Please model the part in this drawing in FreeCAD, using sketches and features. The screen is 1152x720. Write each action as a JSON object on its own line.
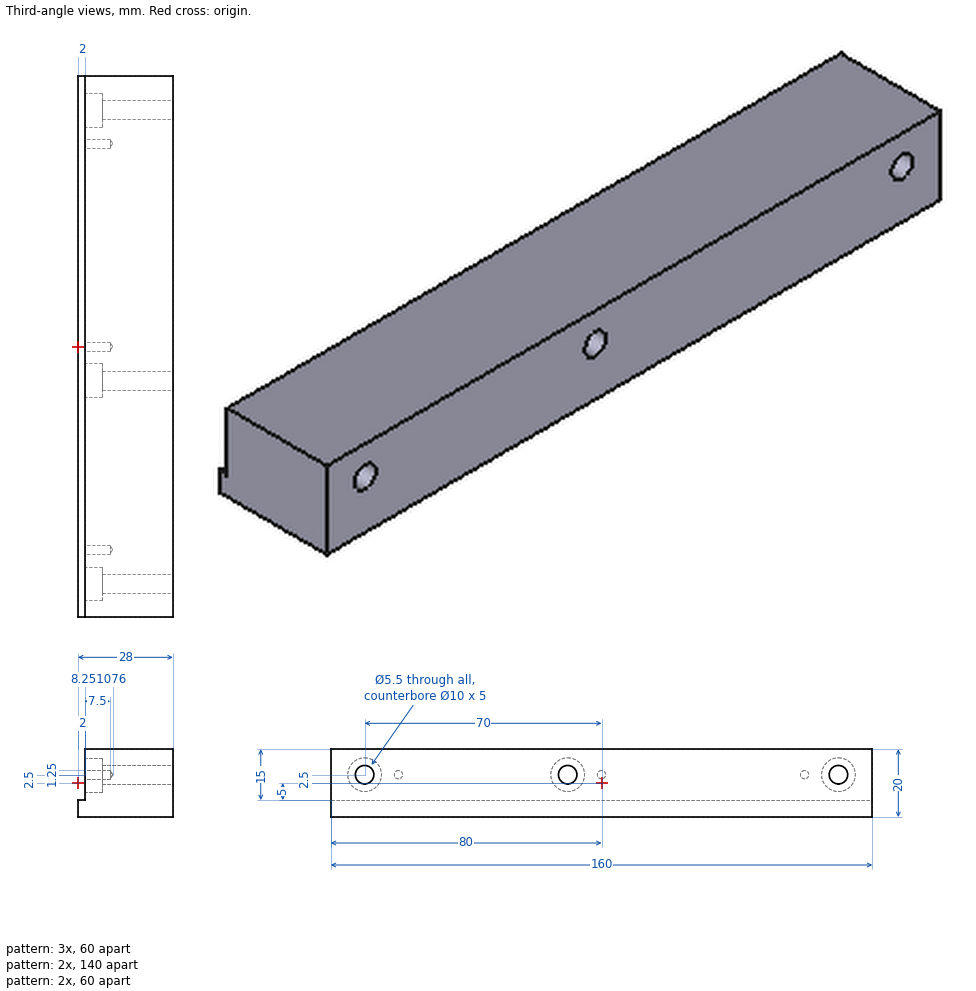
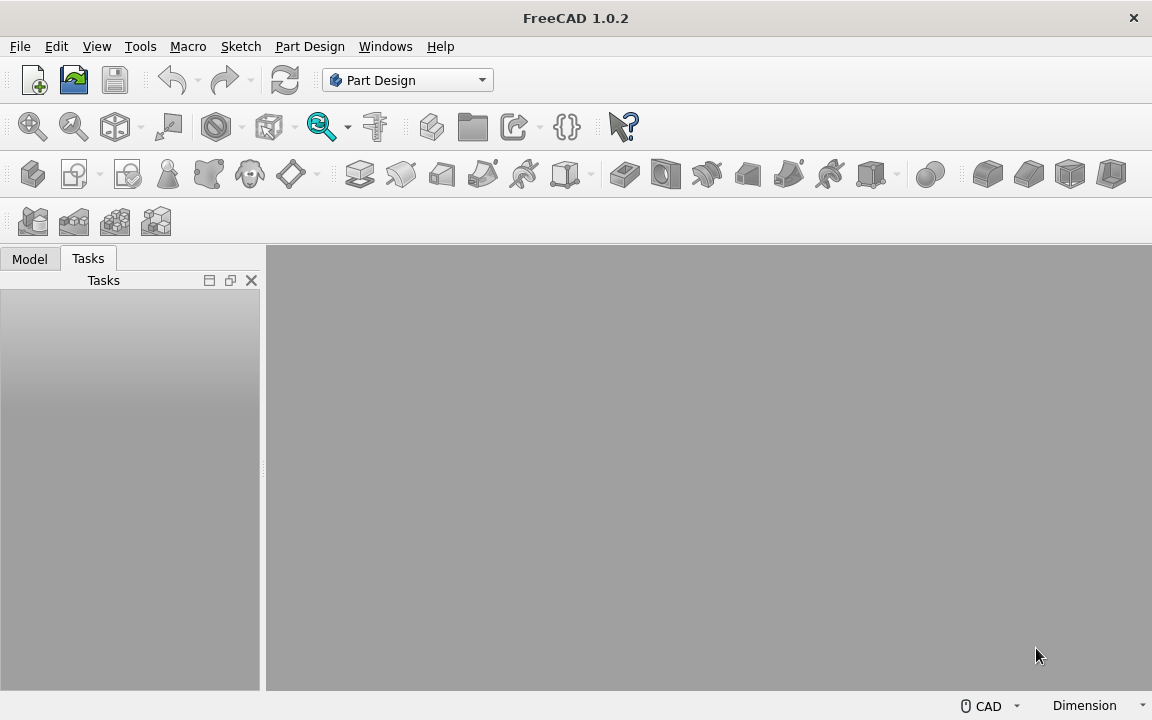
{"action": "left_click", "coordinate": [33, 80]}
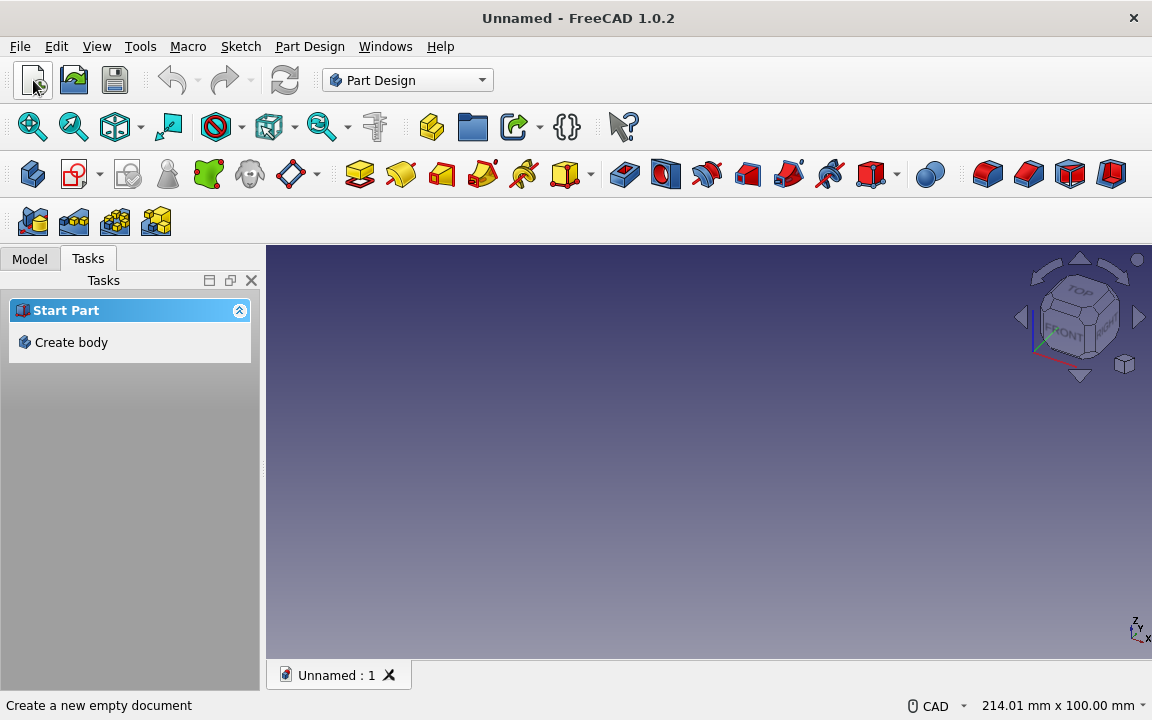
{"action": "left_click", "coordinate": [74, 174]}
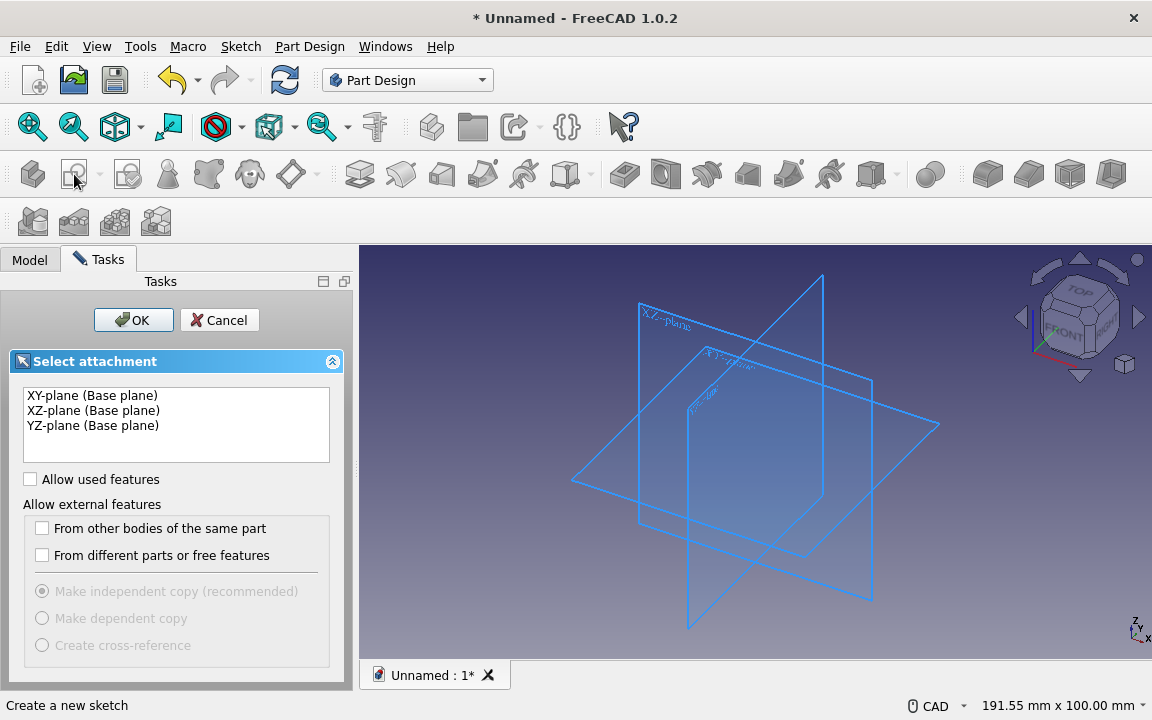
{"action": "left_click", "coordinate": [84, 426]}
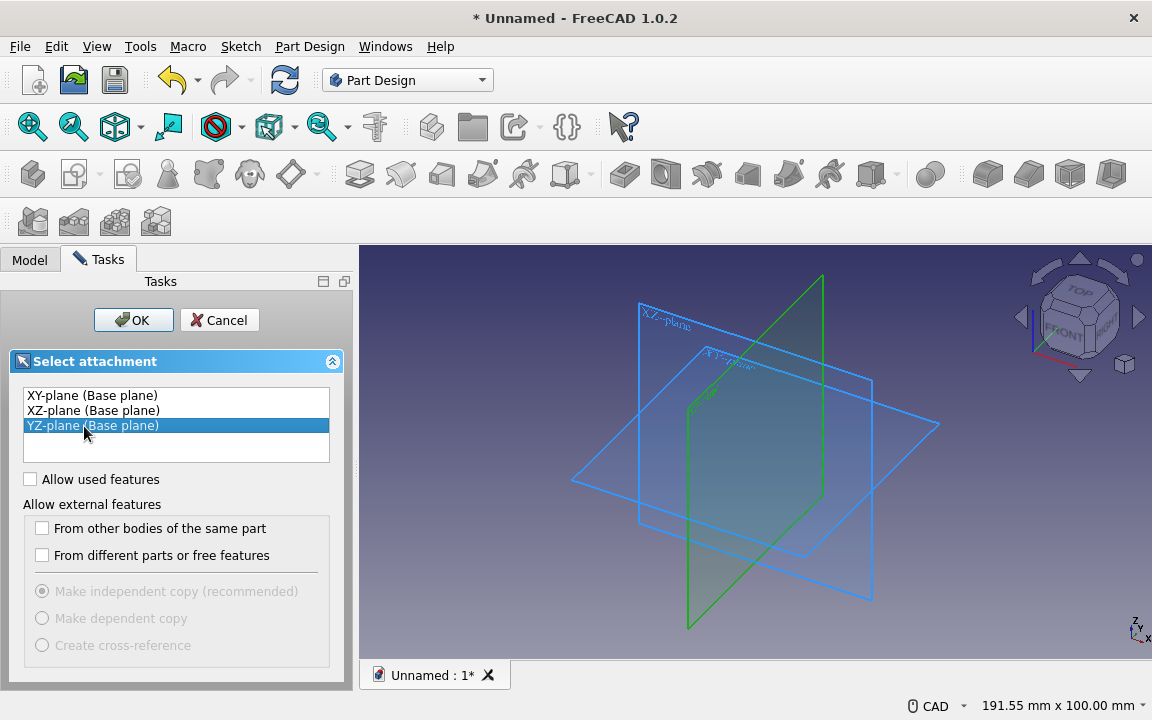
{"action": "left_click", "coordinate": [134, 320]}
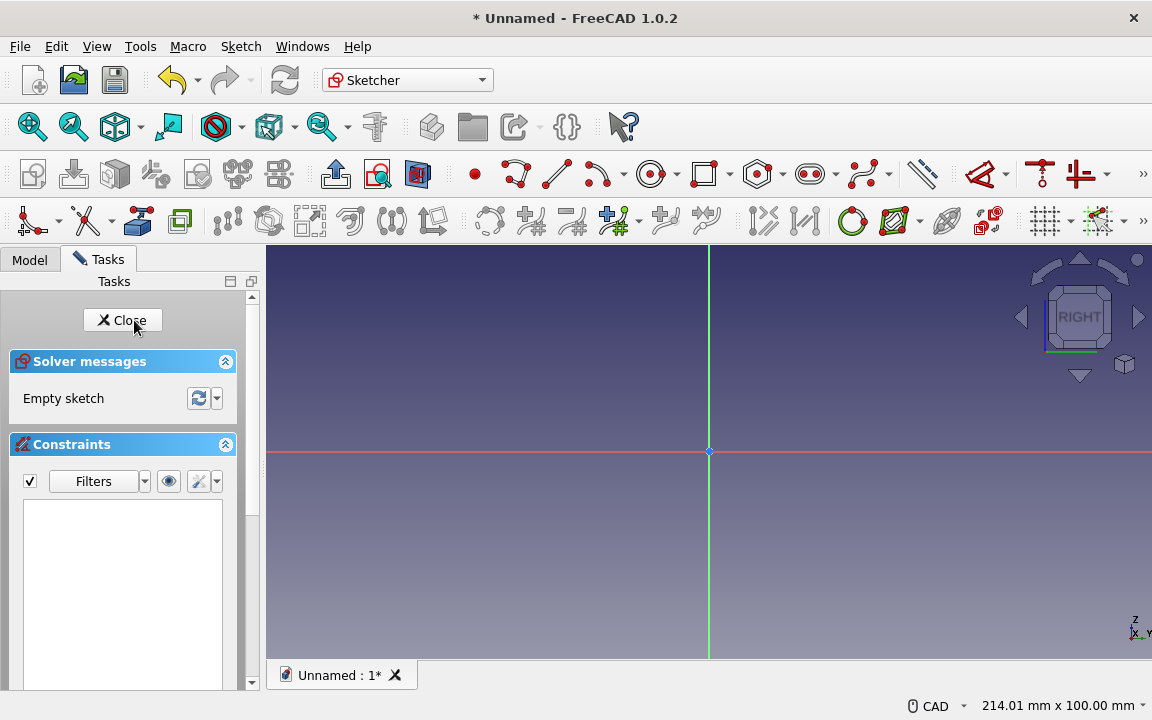
{"action": "scroll", "coordinate": [501, 452], "scroll_direction": "down", "scroll_amount": 2}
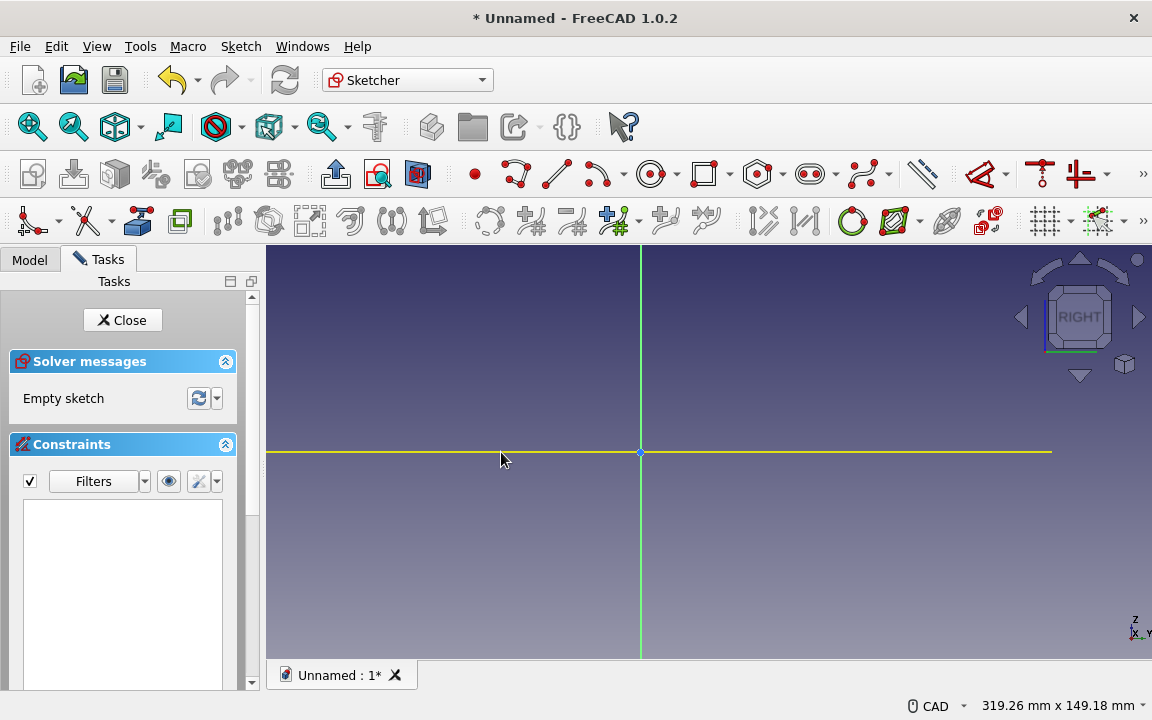
{"action": "key", "text": "g v"}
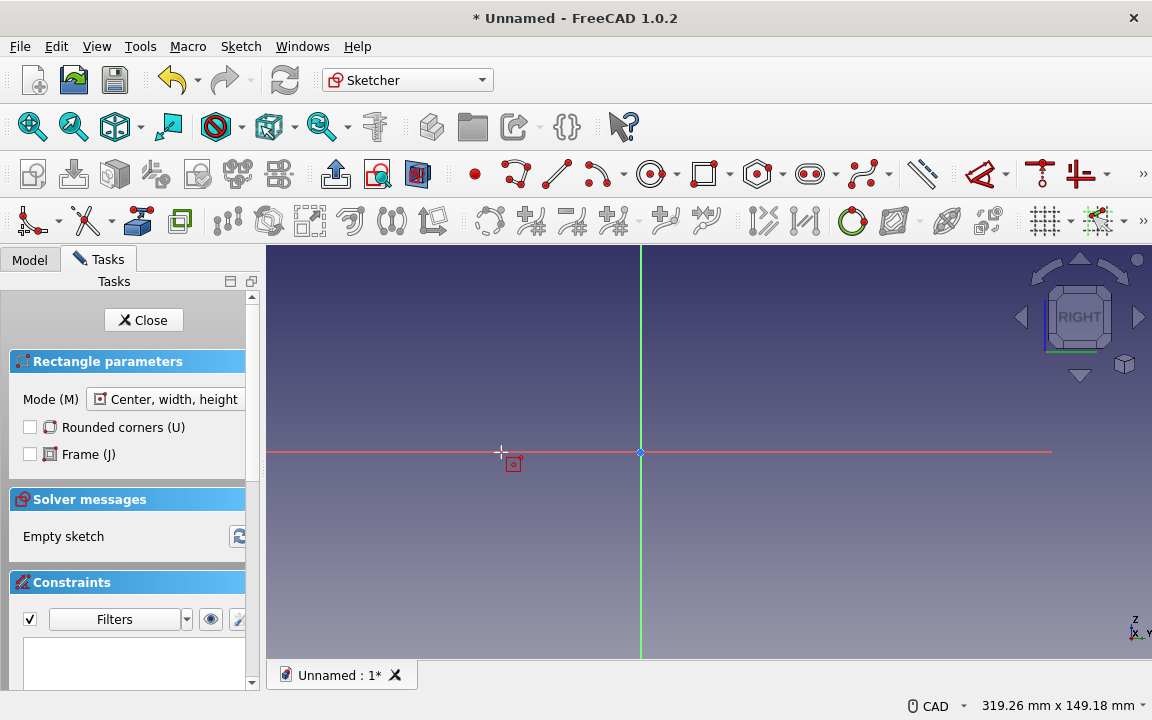
{"action": "left_click", "coordinate": [641, 452]}
{"action": "left_click", "coordinate": [863, 424]}
{"action": "key", "text": "Escape"}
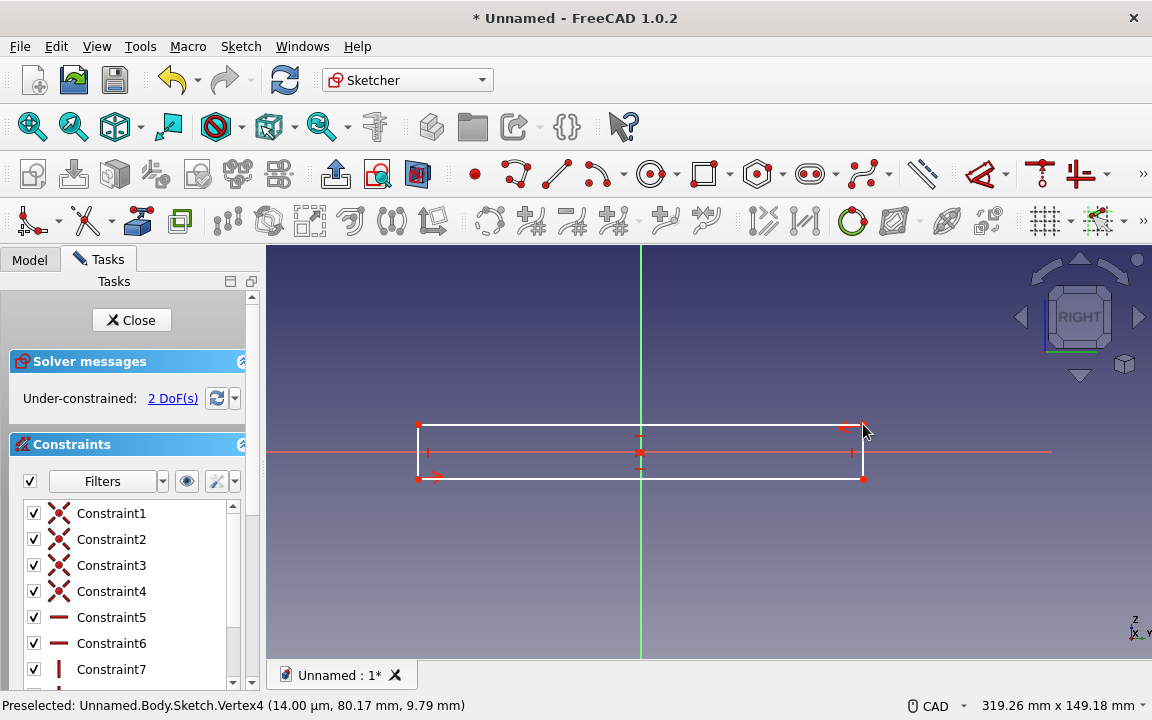
{"action": "key", "text": "d"}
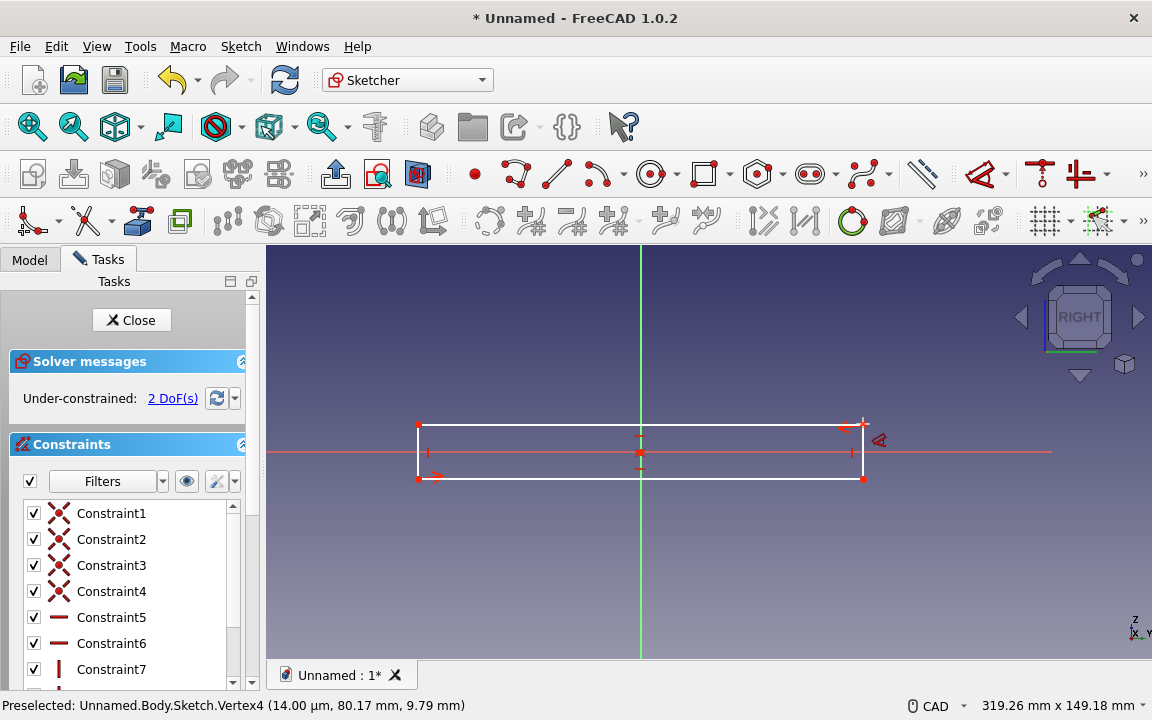
{"action": "scroll", "coordinate": [863, 463], "scroll_direction": "up", "scroll_amount": 2}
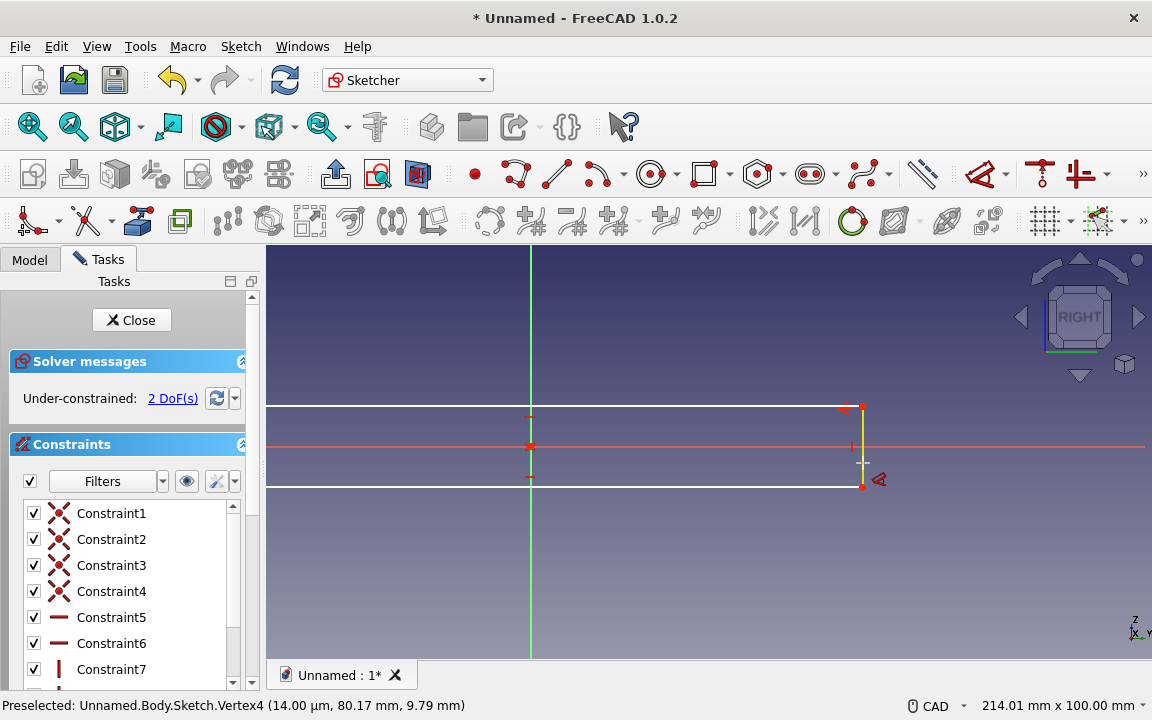
{"action": "left_click", "coordinate": [863, 463]}
{"action": "left_click", "coordinate": [897, 428]}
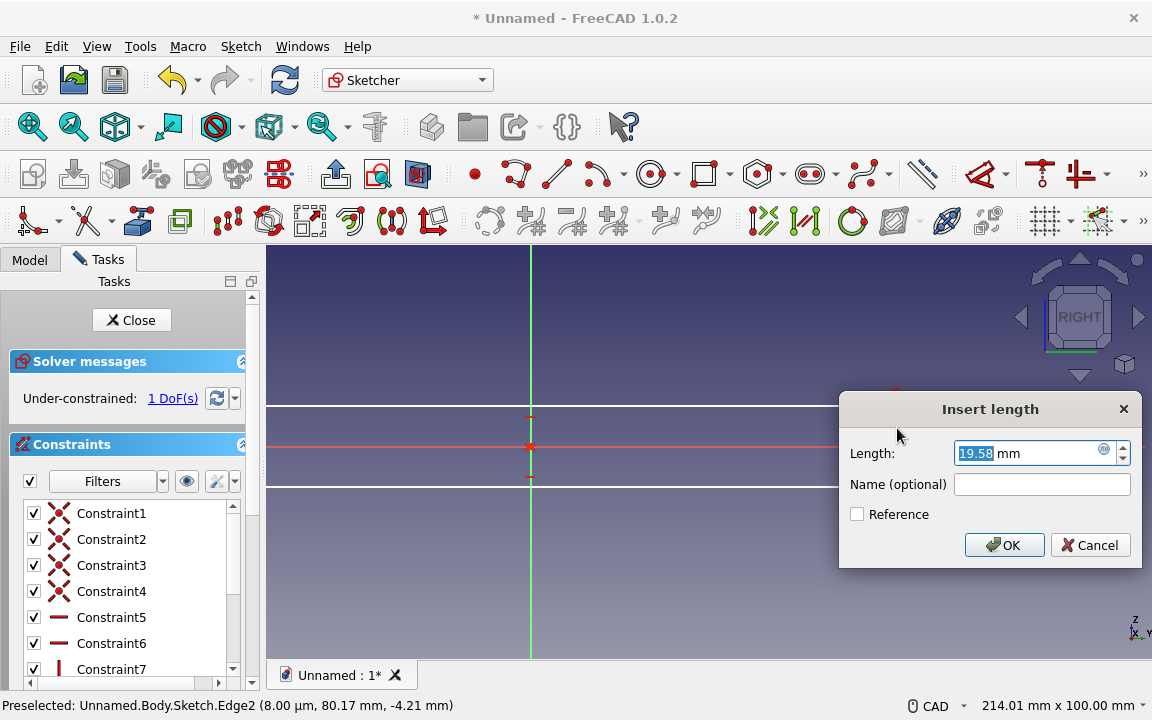
{"action": "type", "text": "20"}
{"action": "key", "text": "Return"}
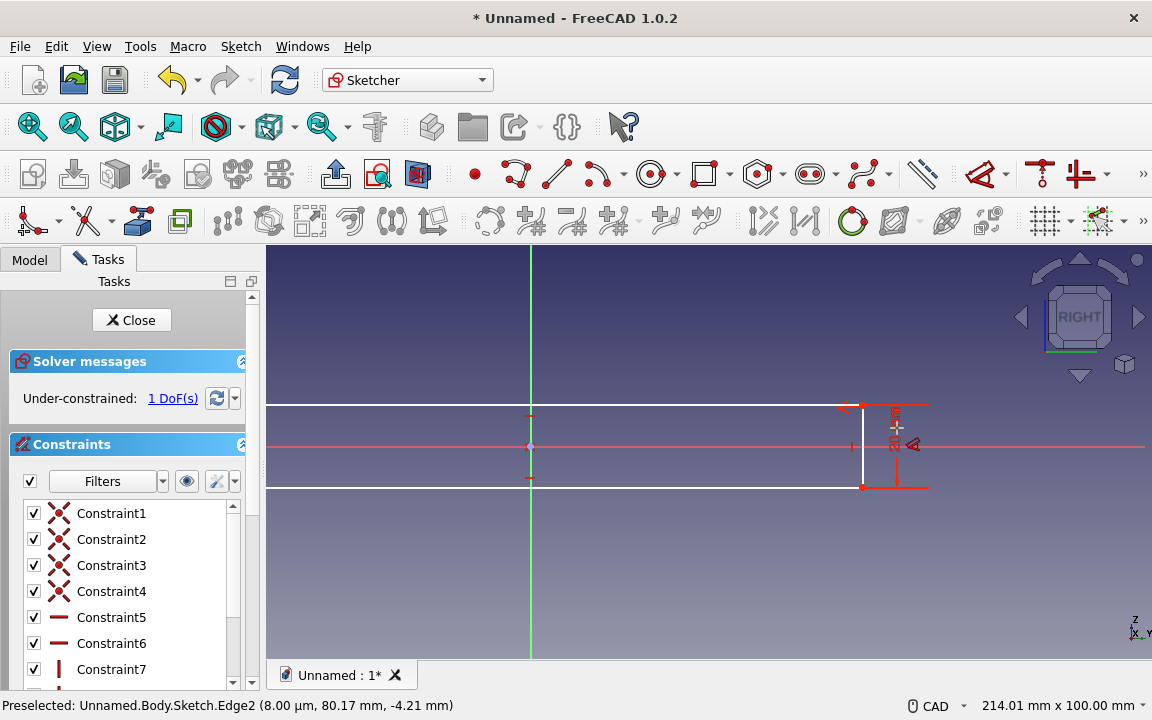
{"action": "left_click", "coordinate": [398, 488]}
{"action": "left_click", "coordinate": [578, 522]}